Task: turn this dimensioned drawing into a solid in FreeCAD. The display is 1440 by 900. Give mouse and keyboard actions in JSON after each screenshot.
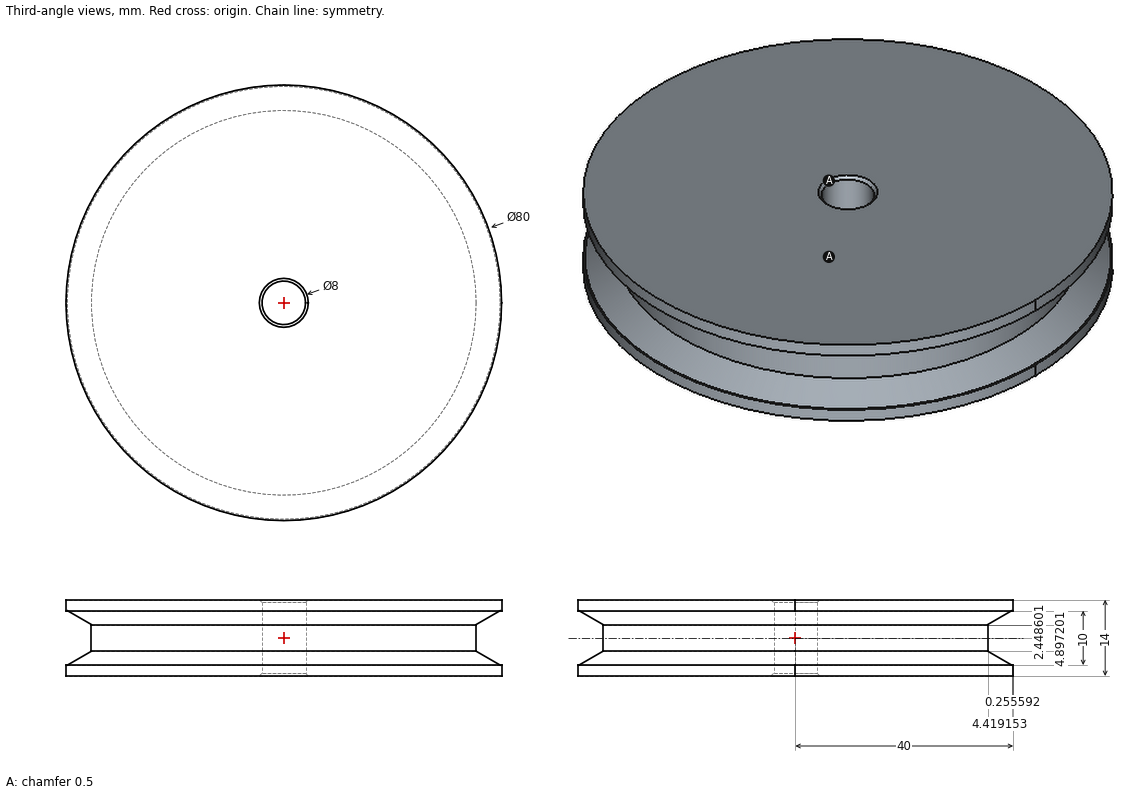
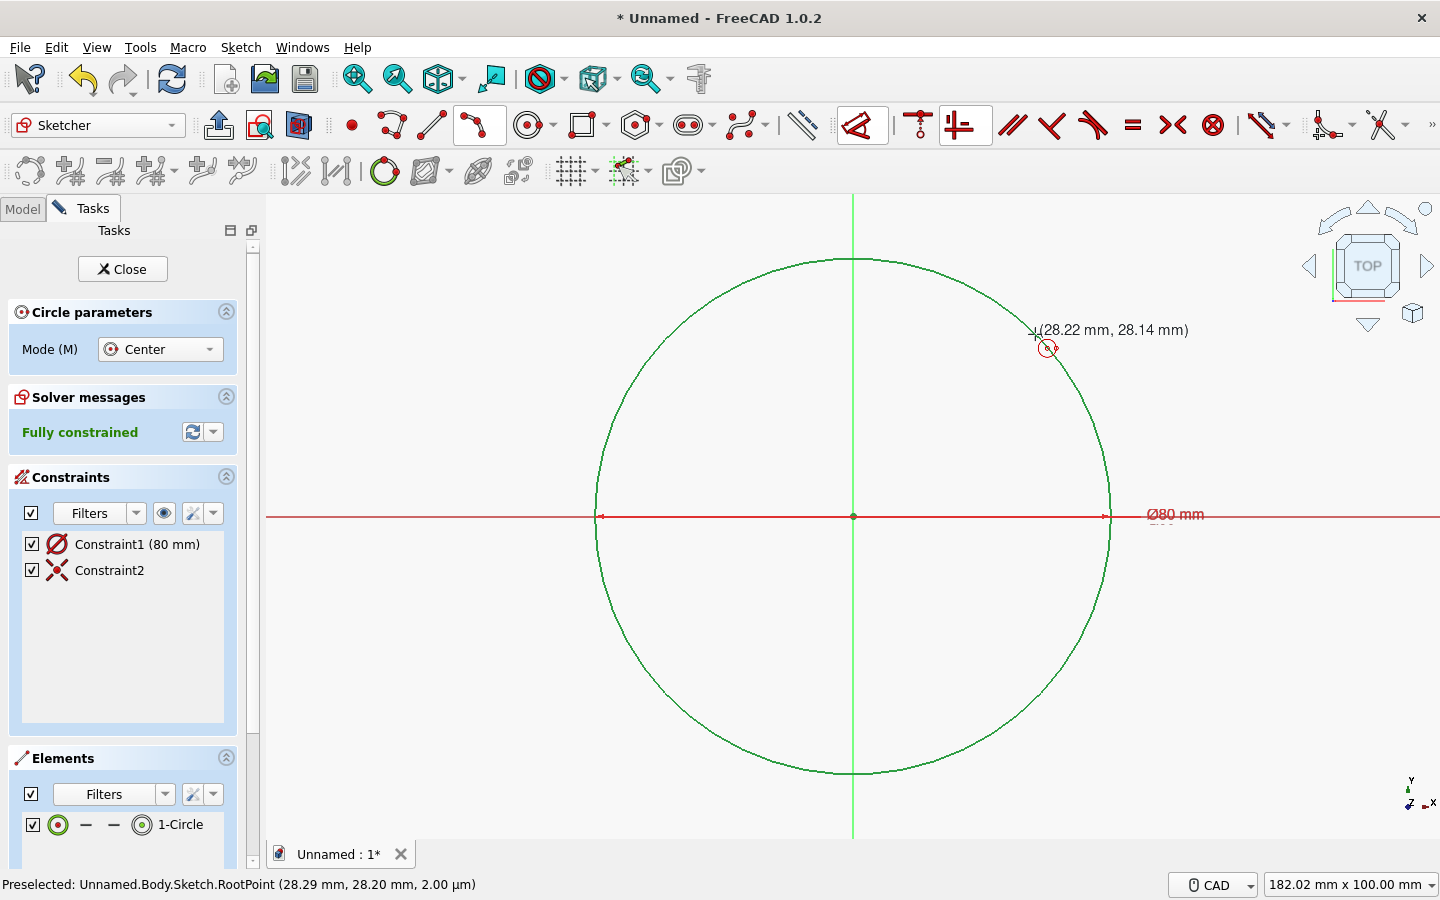
{"action": "left_click", "coordinate": [853, 516]}
{"action": "mouse_move", "coordinate": [871, 498]}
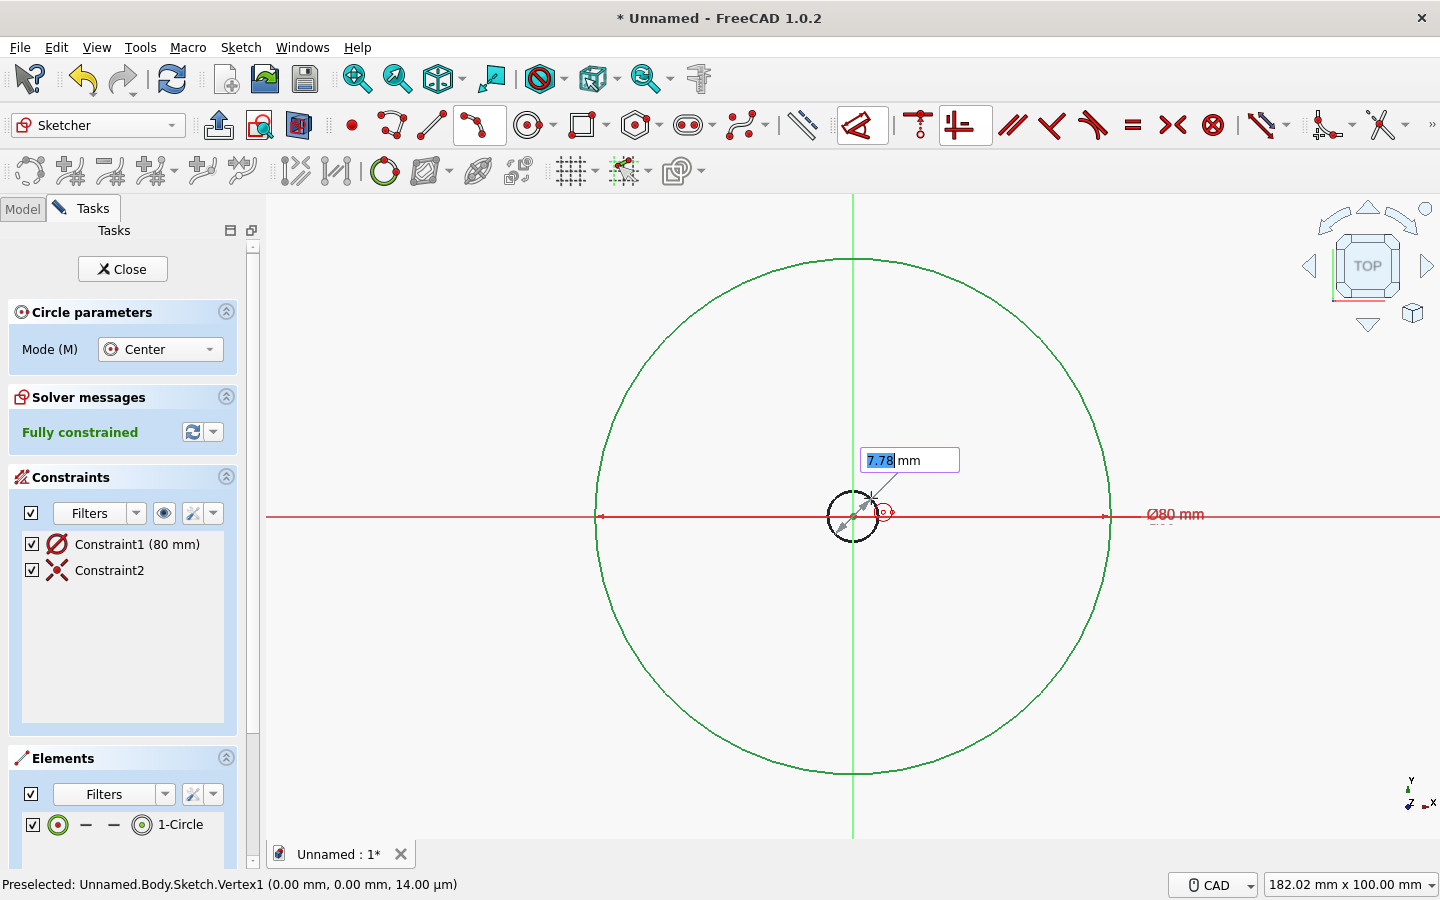
{"action": "type", "text": "8"}
{"action": "key", "text": "Return"}
{"action": "key", "text": "Escape"}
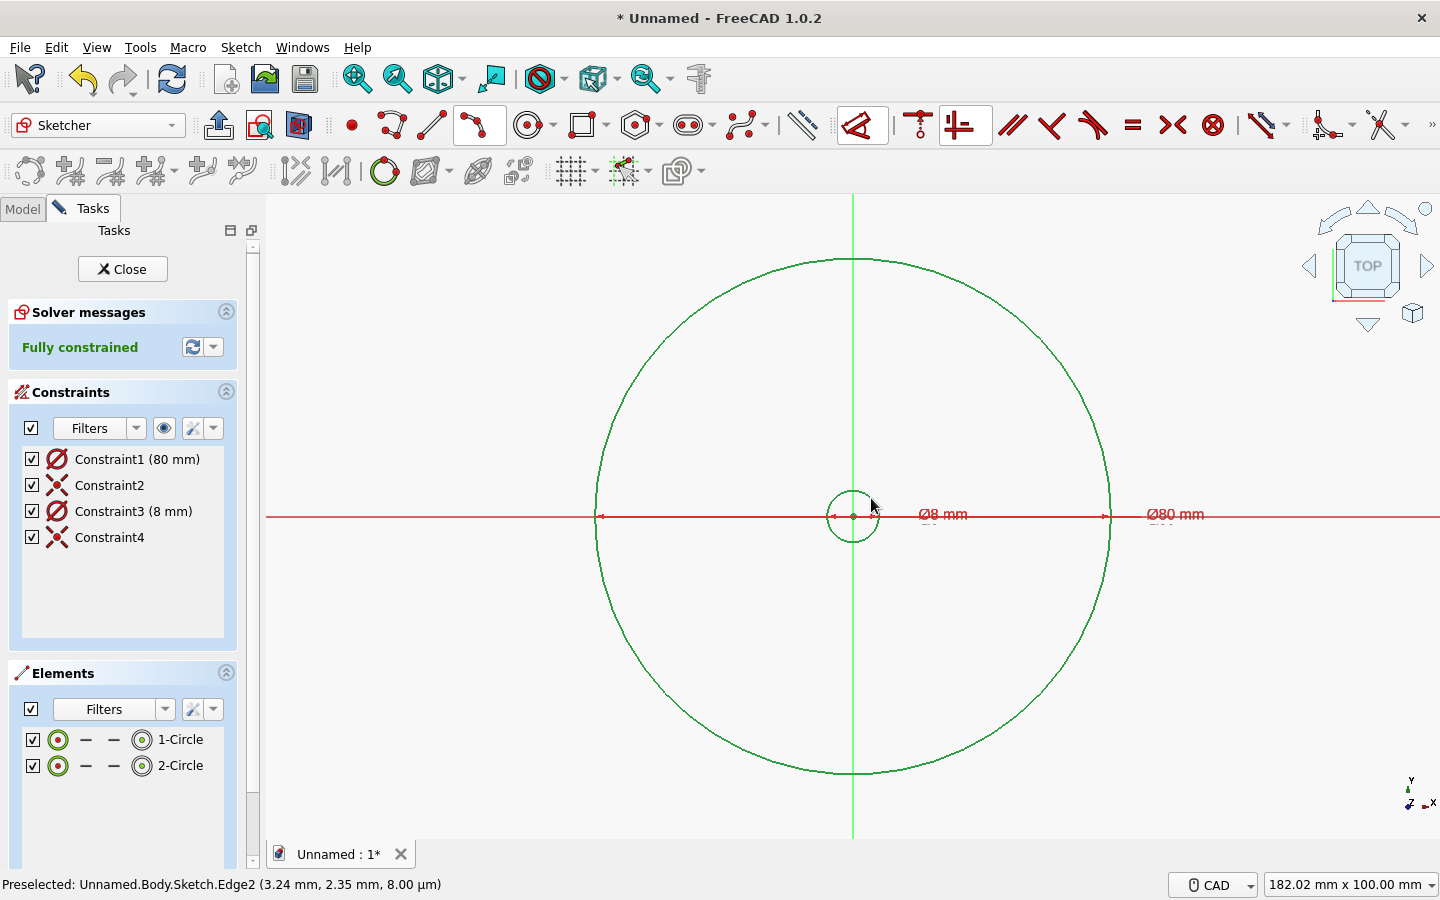
{"action": "left_click", "coordinate": [123, 269]}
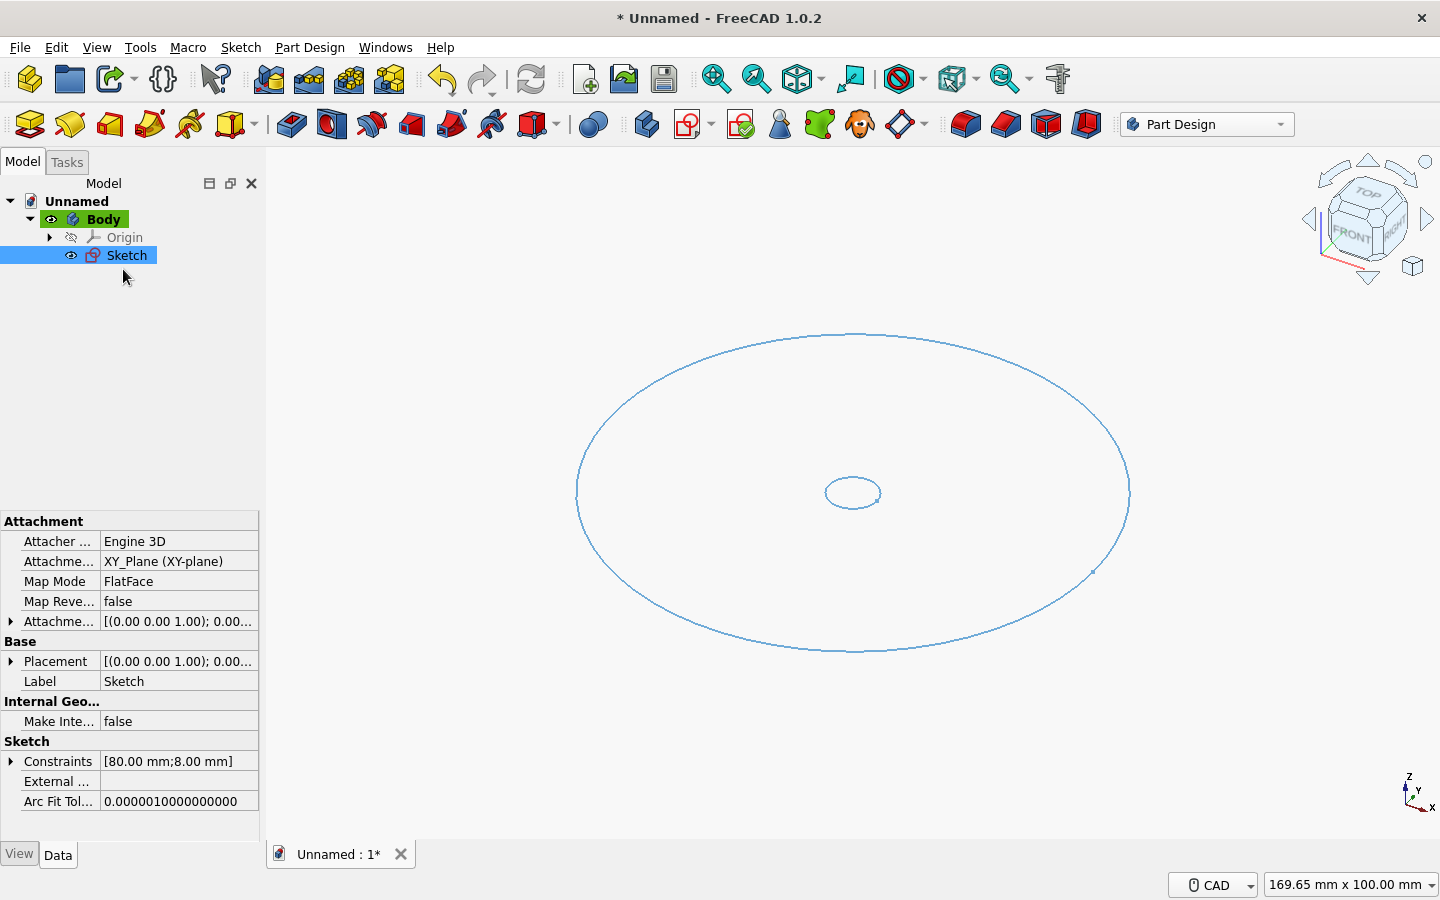
{"action": "left_click", "coordinate": [30, 124]}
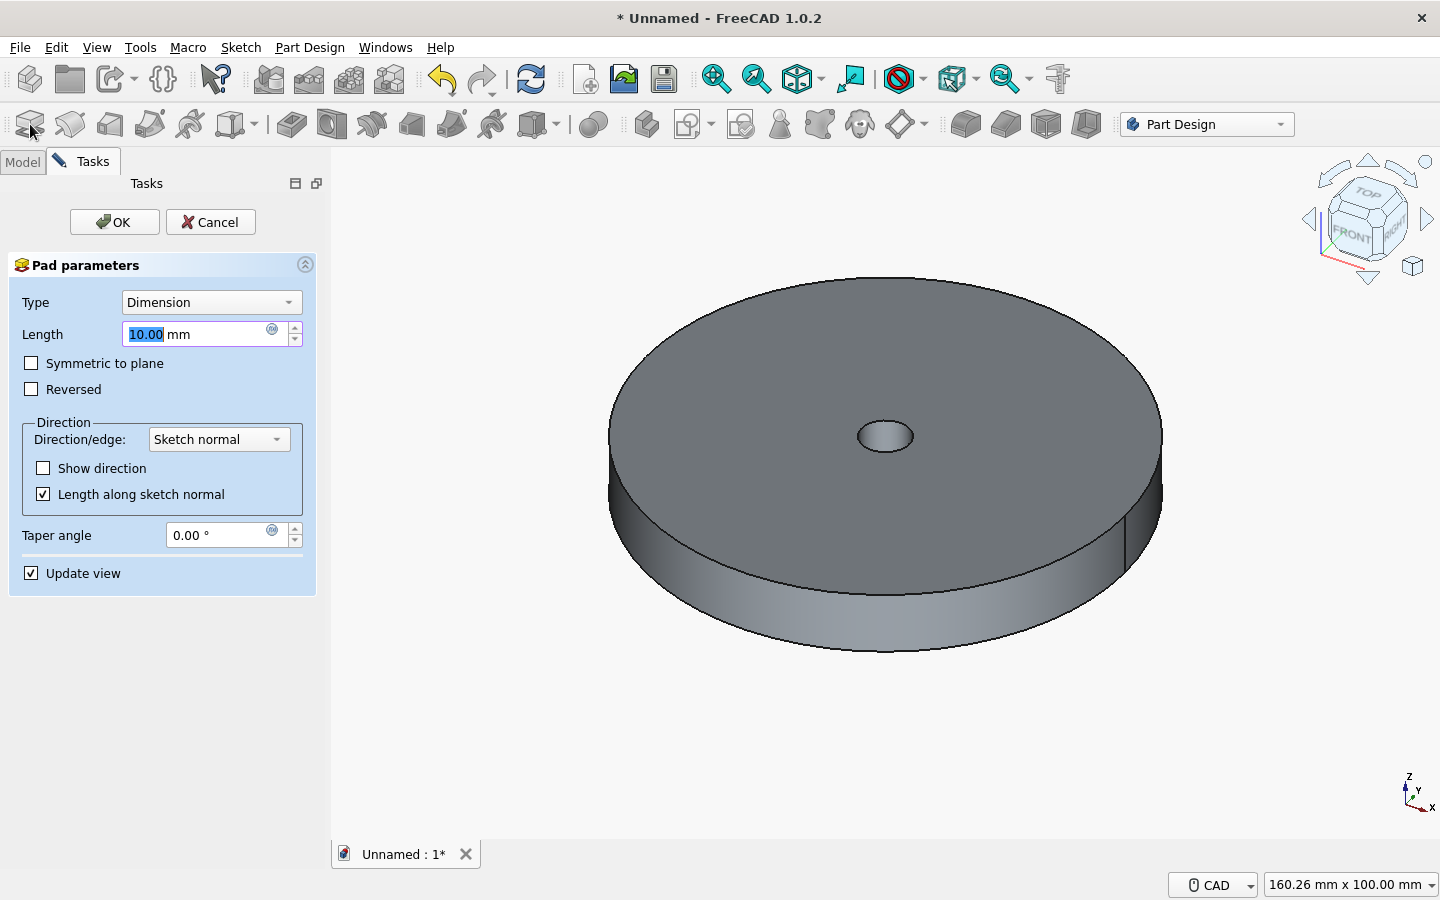
{"action": "type", "text": "14"}
{"action": "key", "text": "Tab"}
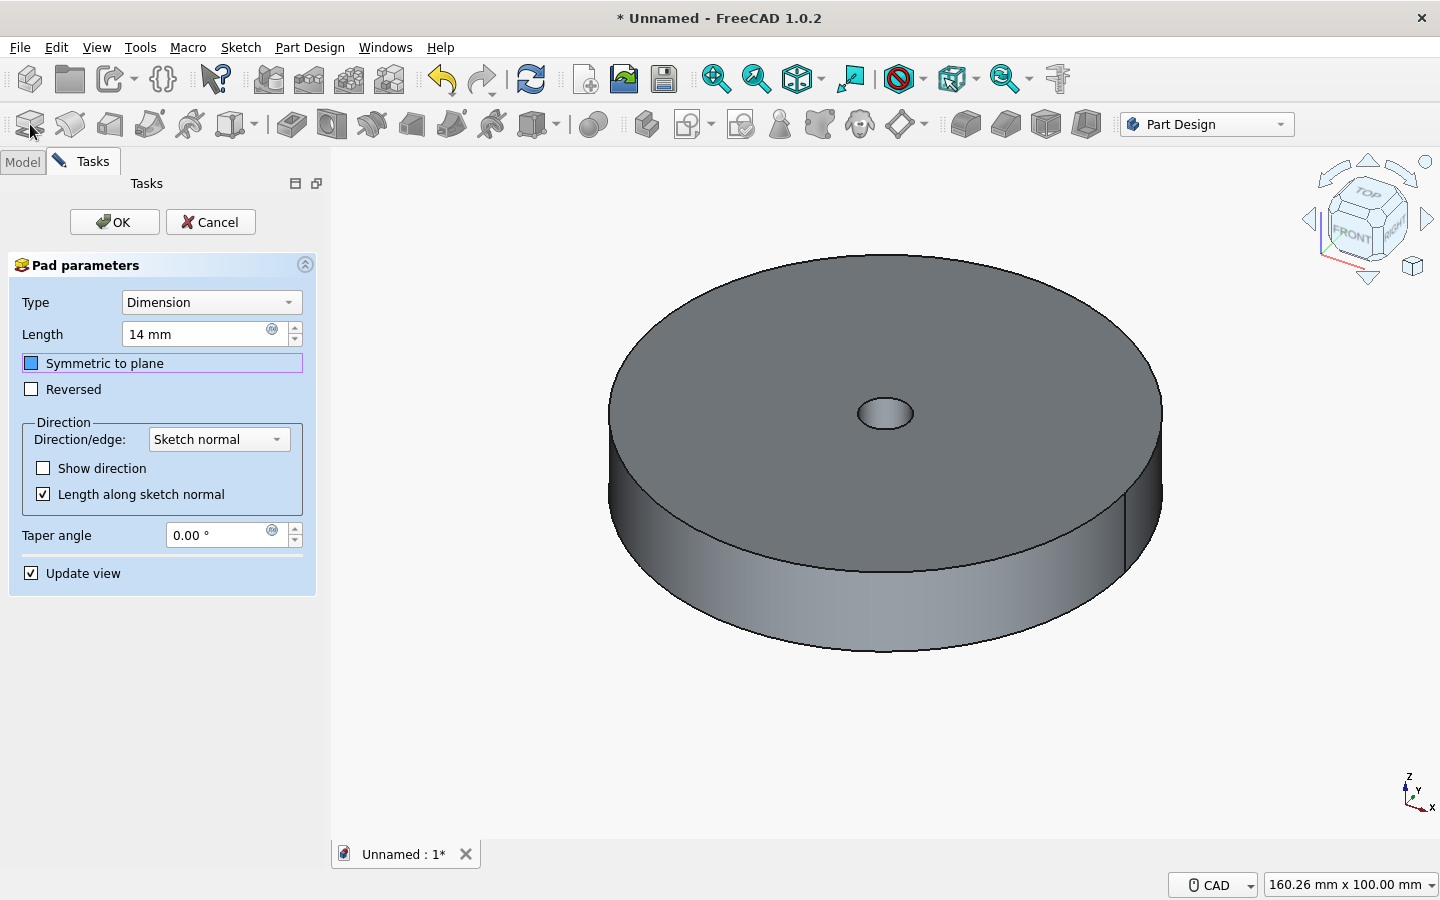
{"action": "left_click", "coordinate": [30, 363]}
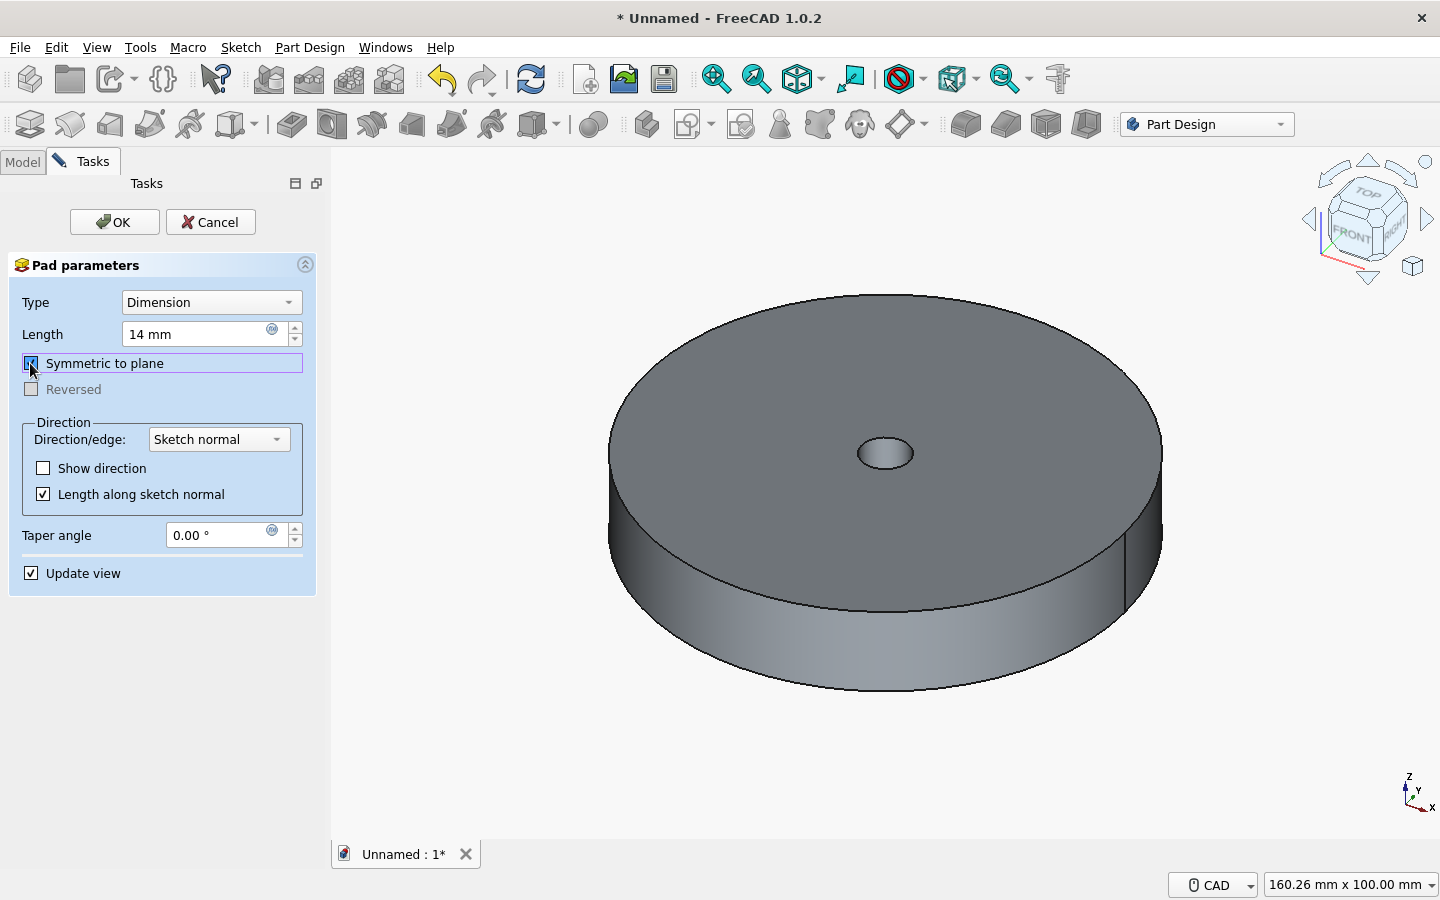
{"action": "left_click", "coordinate": [115, 222]}